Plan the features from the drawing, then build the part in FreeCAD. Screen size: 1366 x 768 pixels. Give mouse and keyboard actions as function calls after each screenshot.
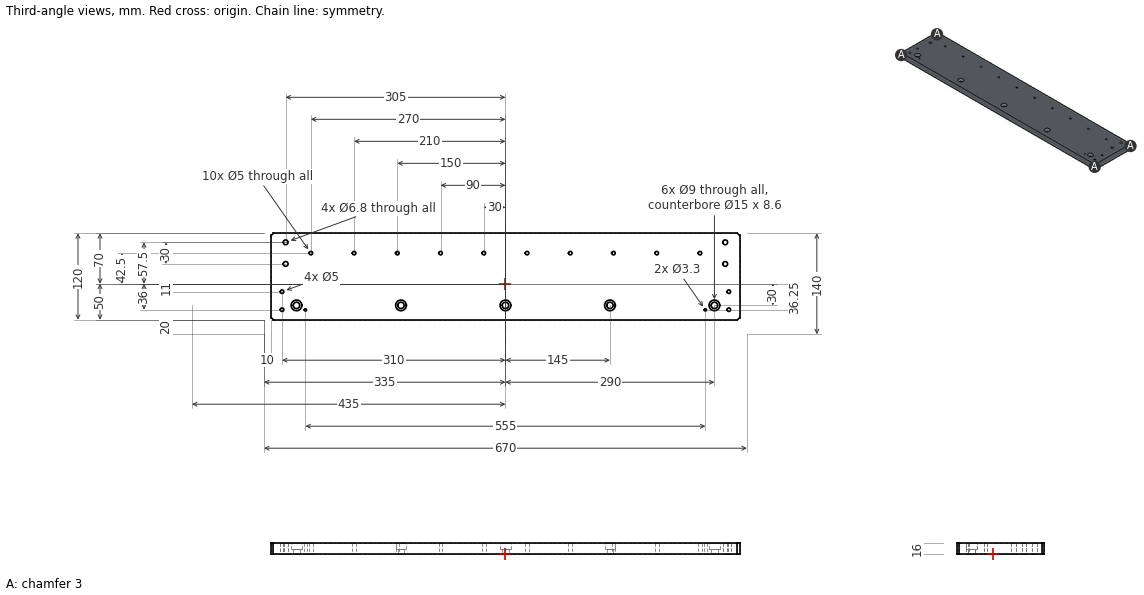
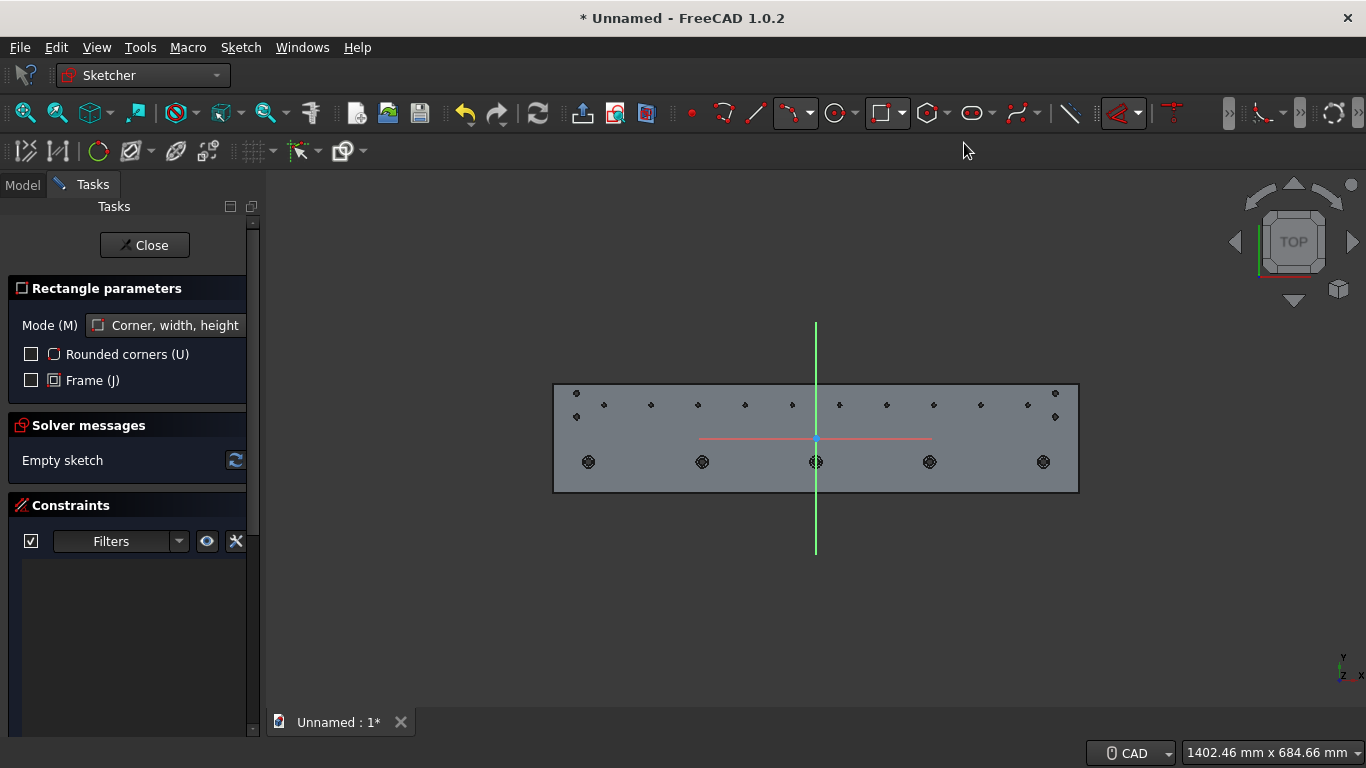
click(553, 478)
click(1079, 493)
key(Escape)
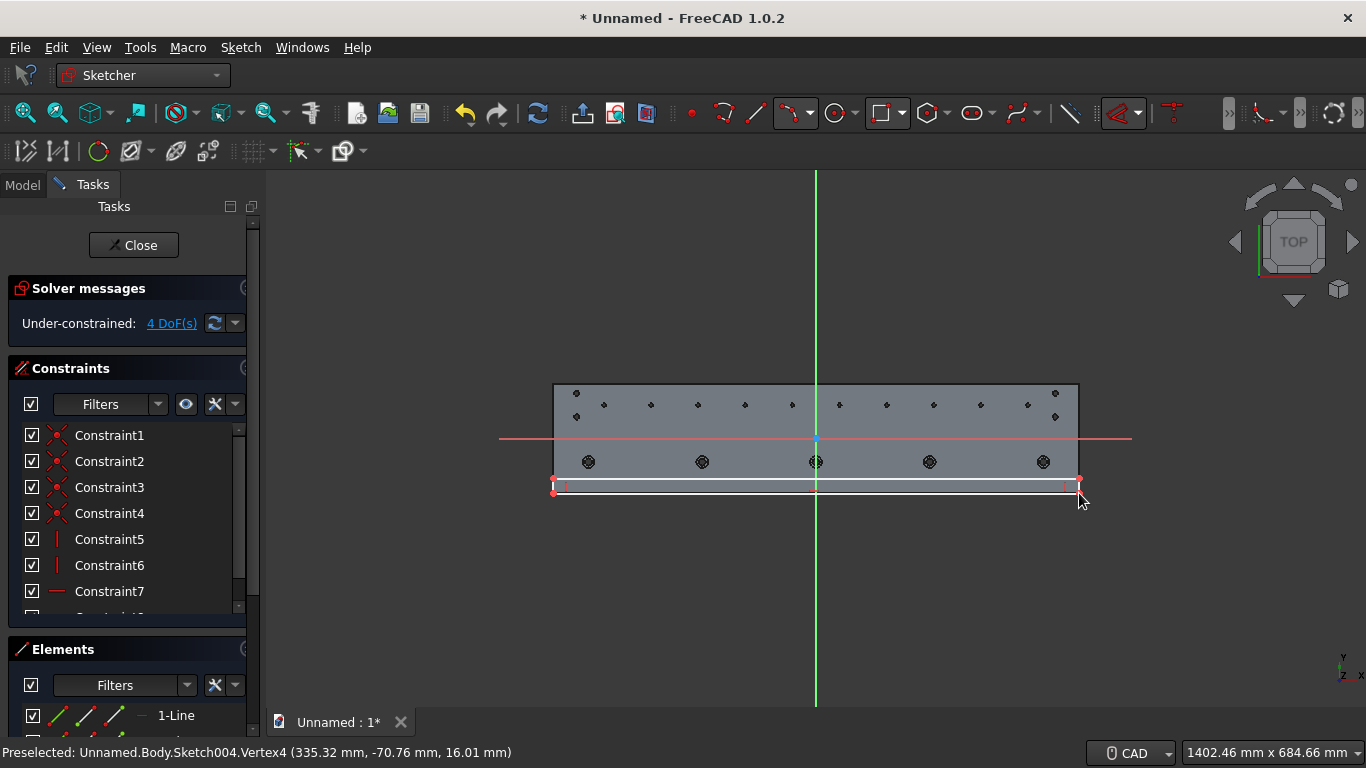
scroll(553, 487, up, 5)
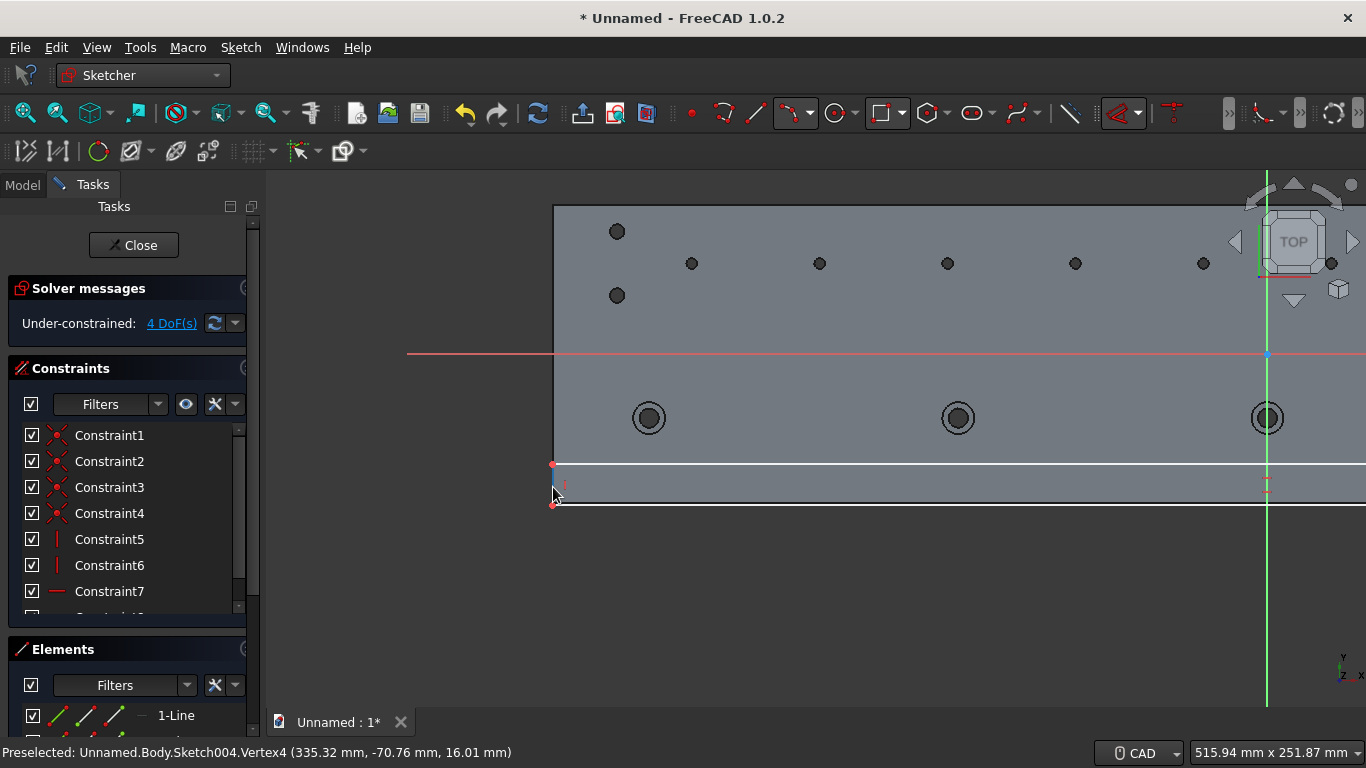
click(553, 485)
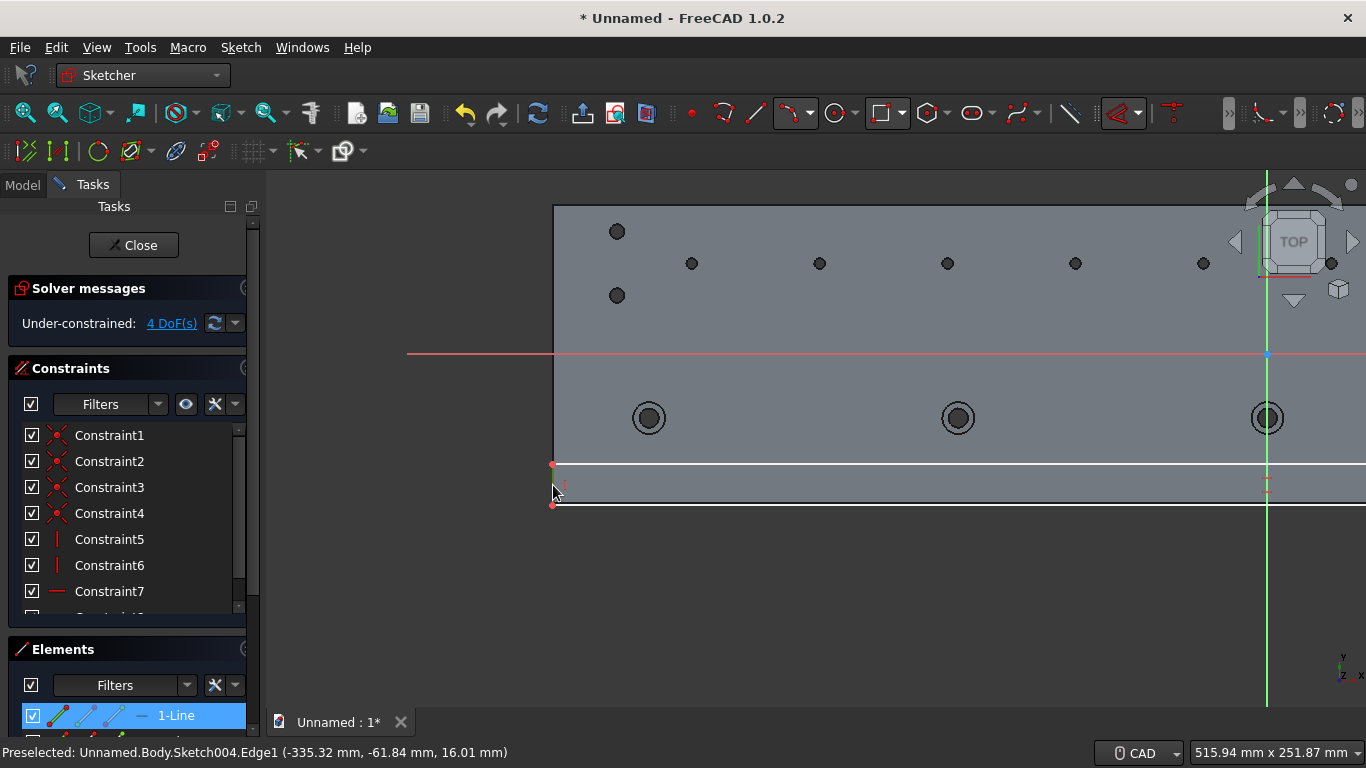
click(1140, 114)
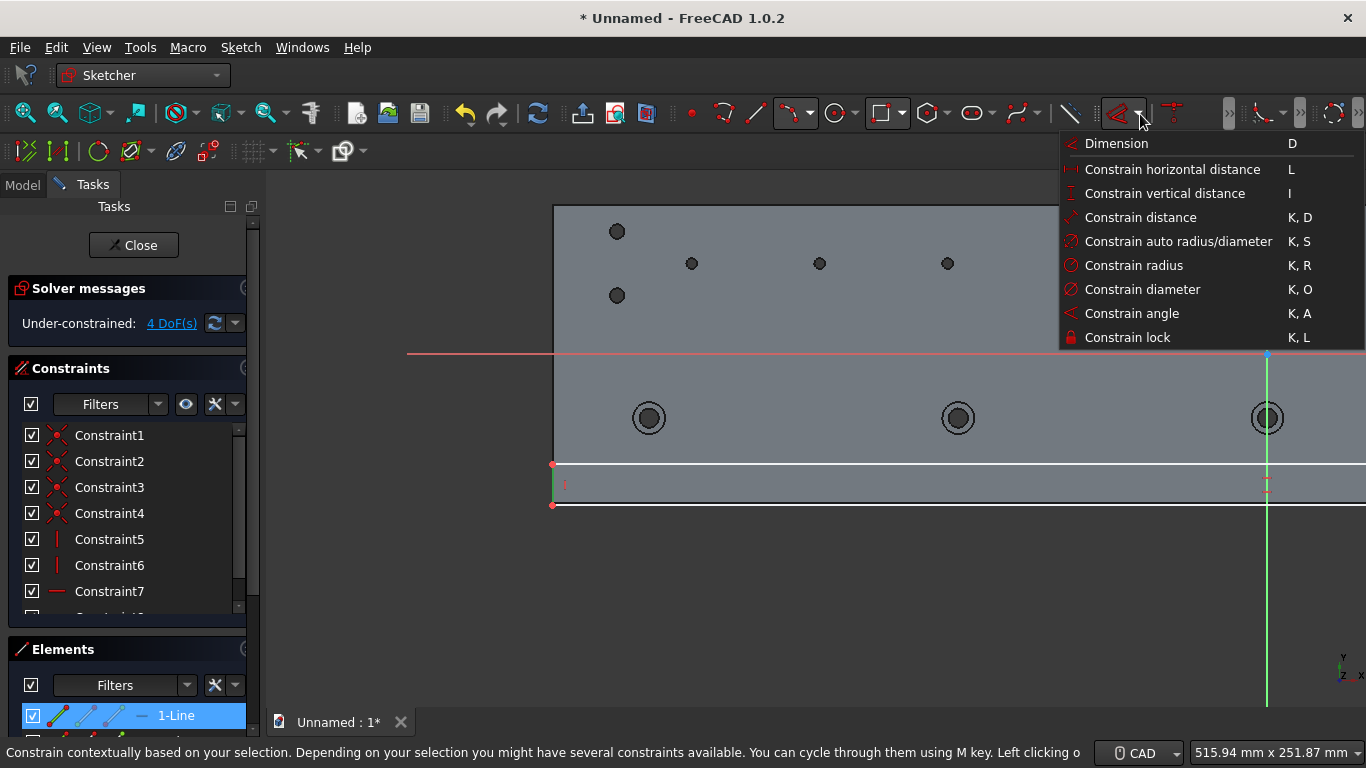
click(1212, 193)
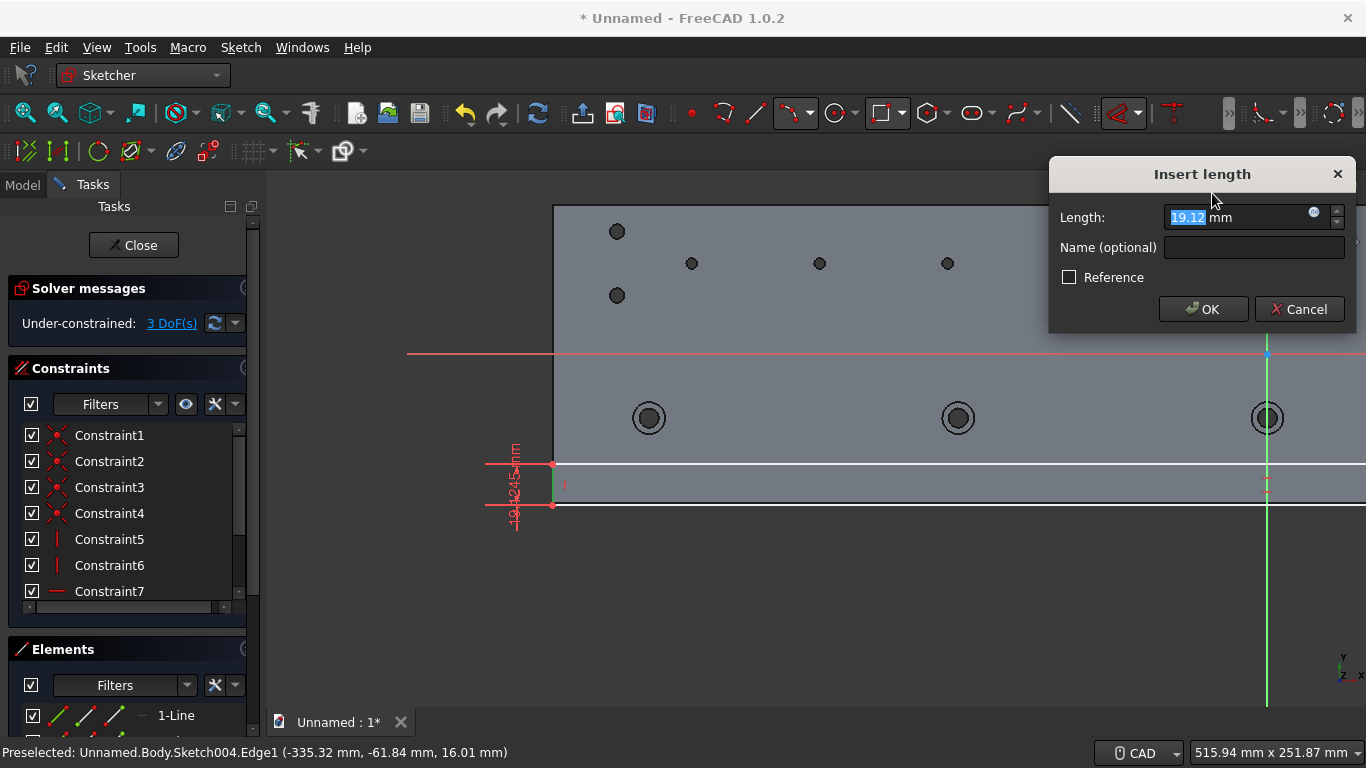
text(20)
key(Return)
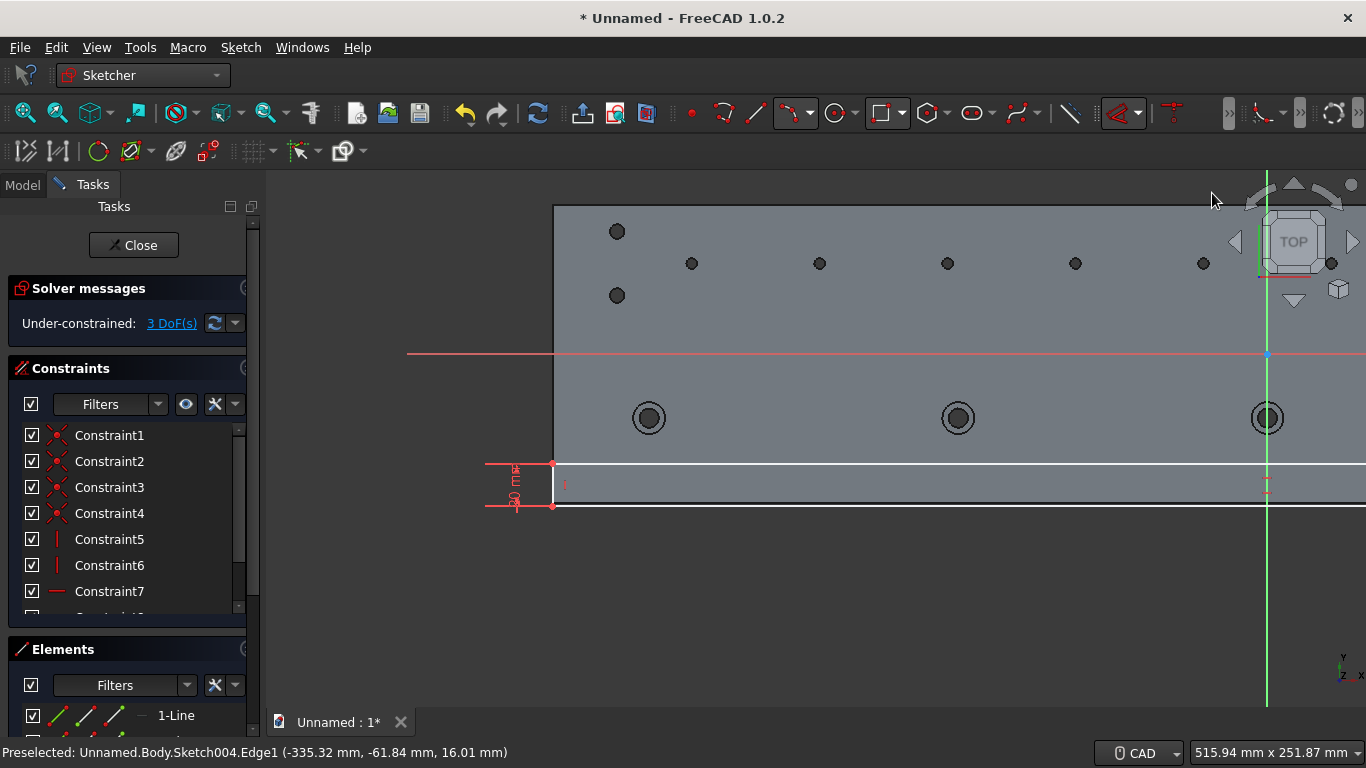
click(981, 506)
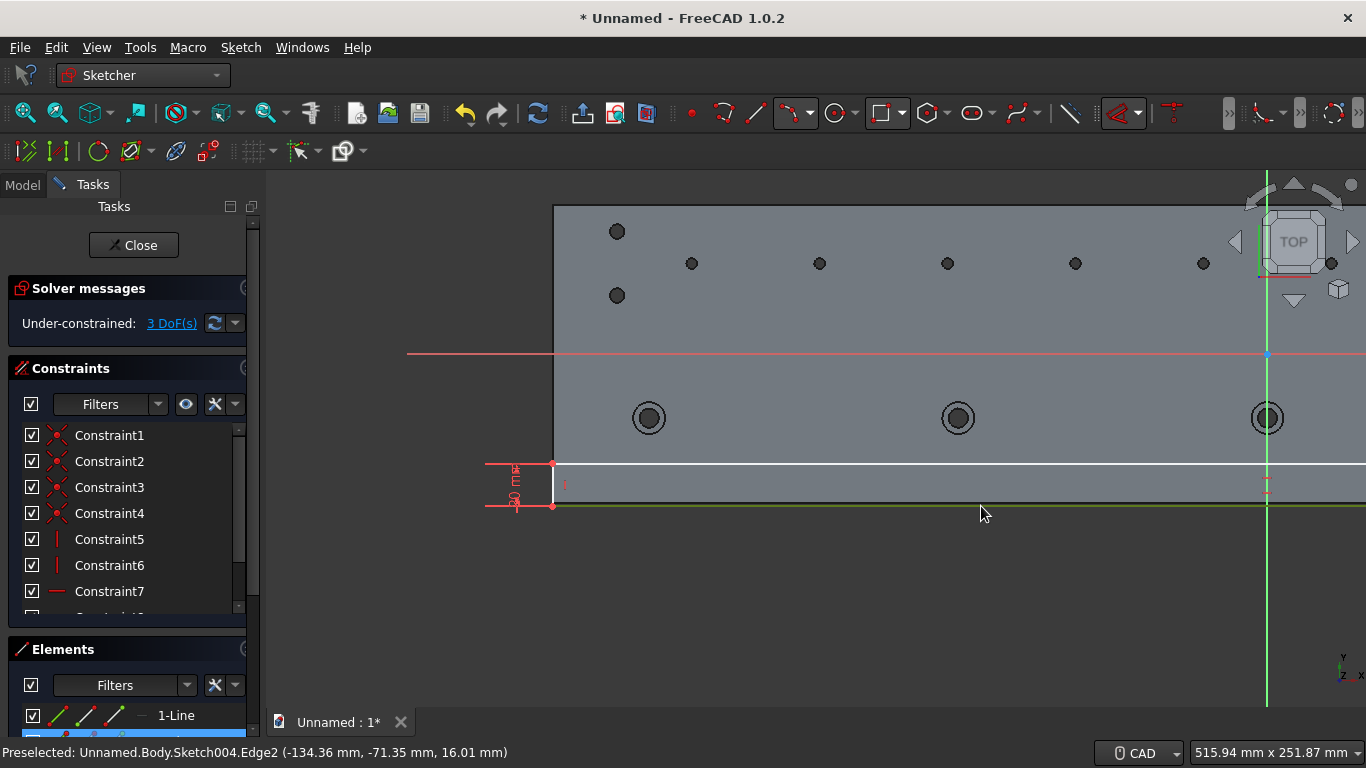
click(1140, 114)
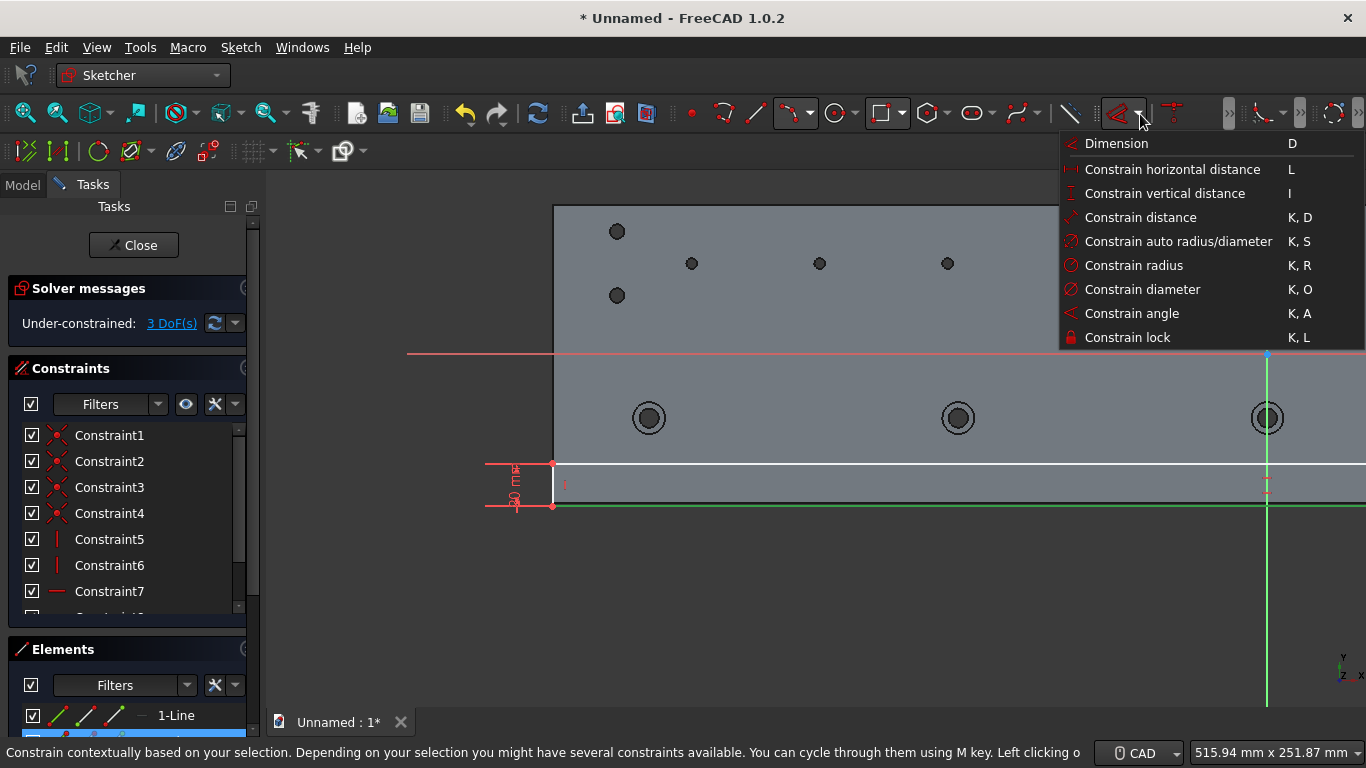
click(1212, 169)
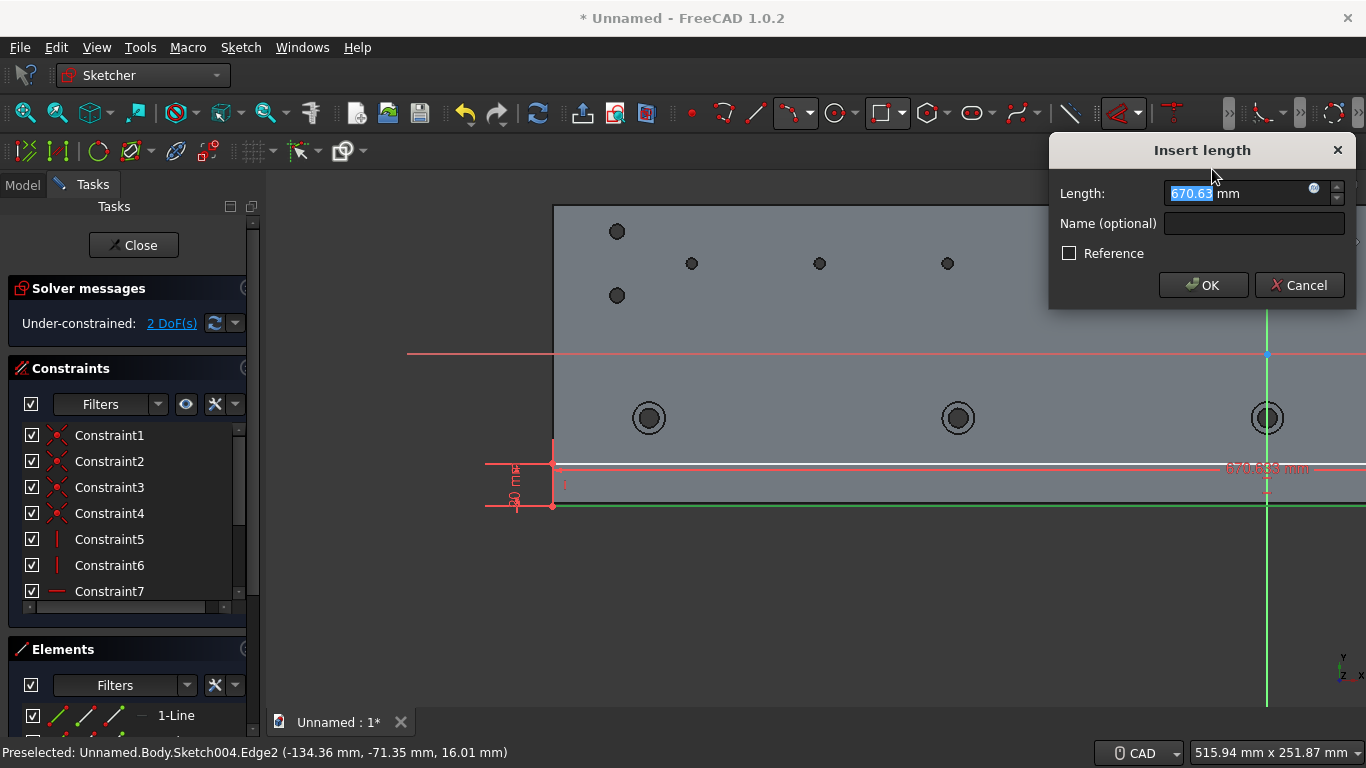
text(670)
key(Return)